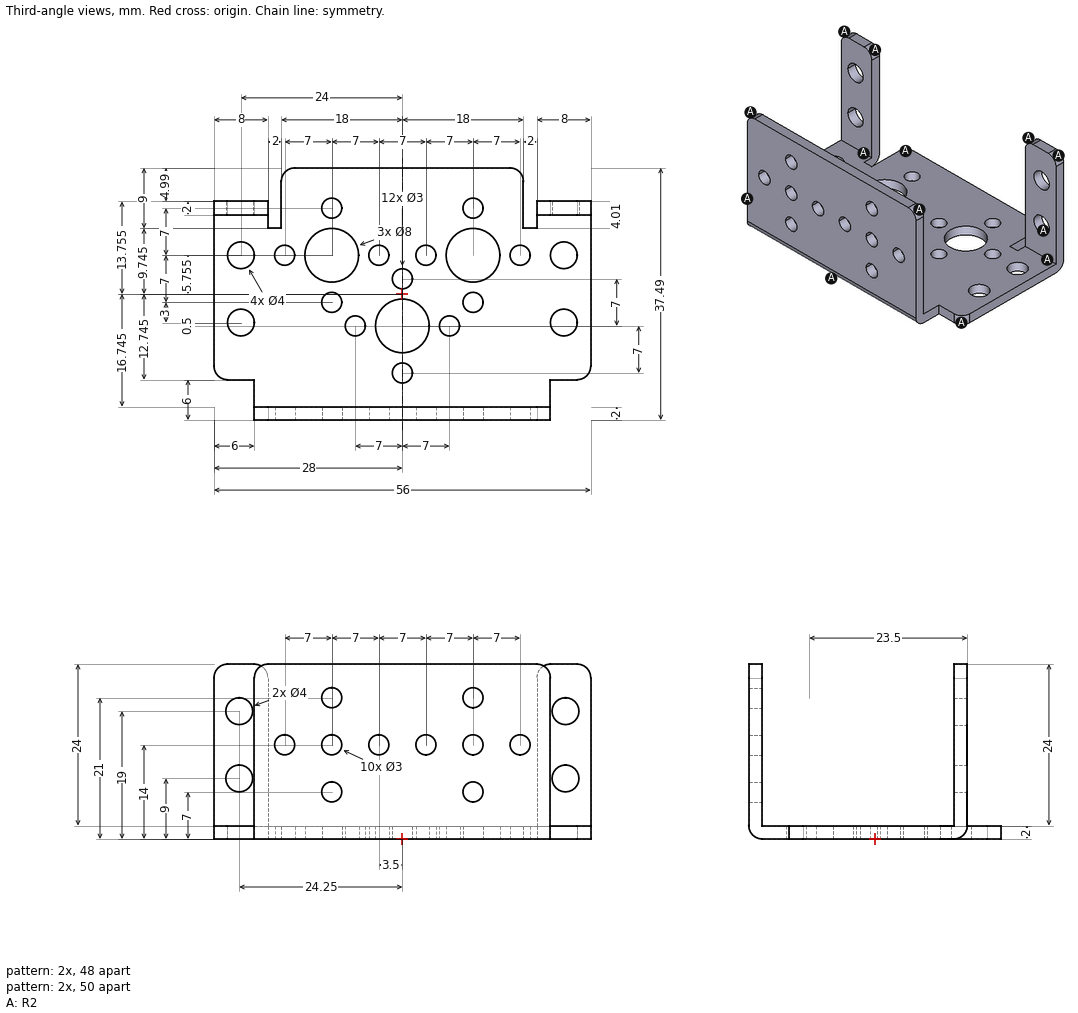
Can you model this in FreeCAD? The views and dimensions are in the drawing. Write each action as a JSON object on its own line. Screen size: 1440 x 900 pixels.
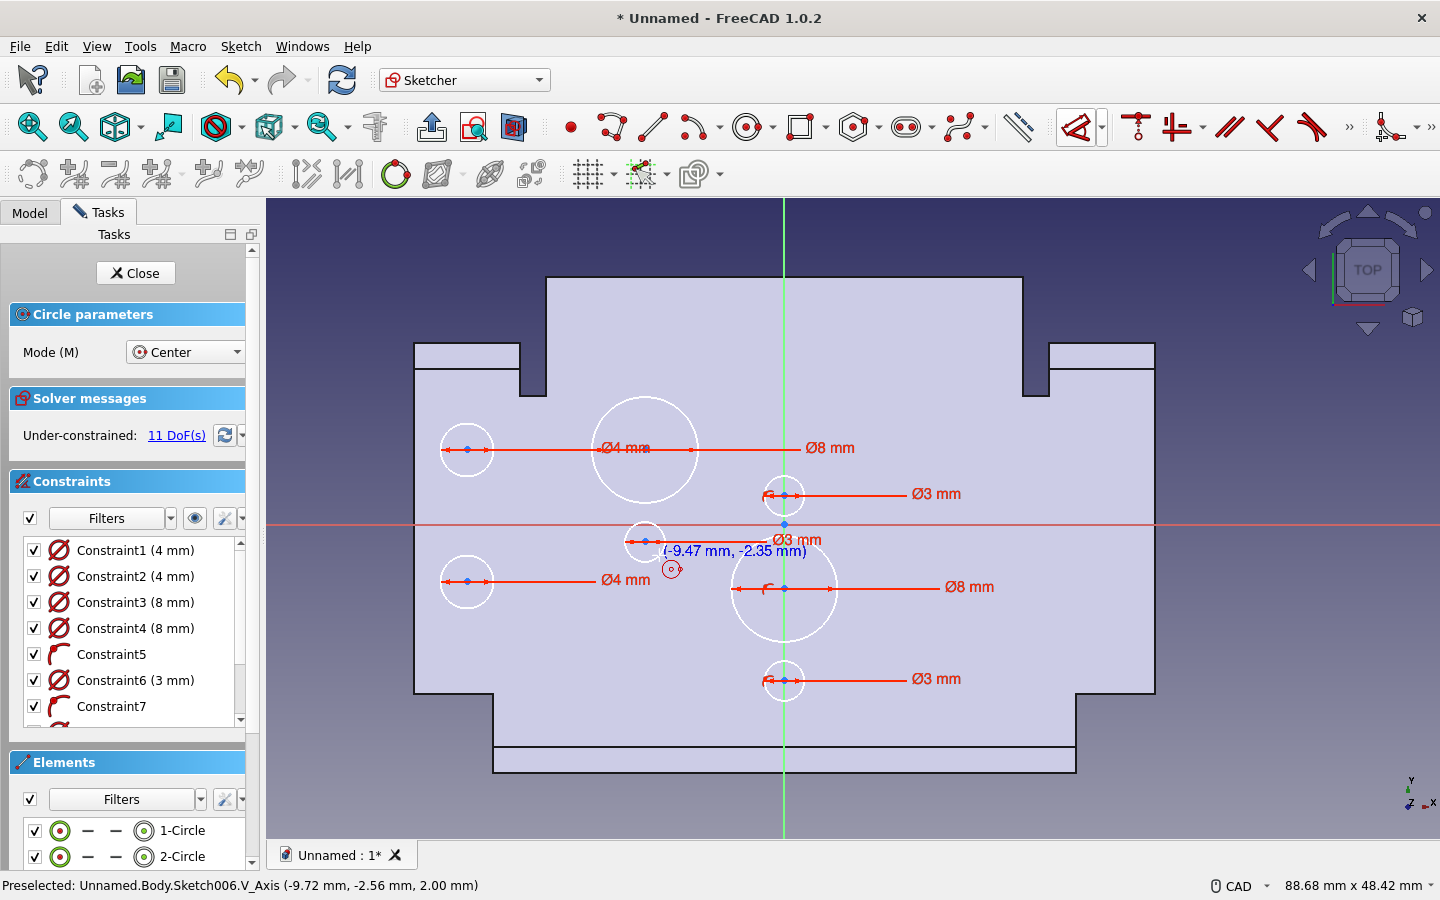
{"action": "left_click", "coordinate": [645, 356]}
{"action": "mouse_move", "coordinate": [659, 342]}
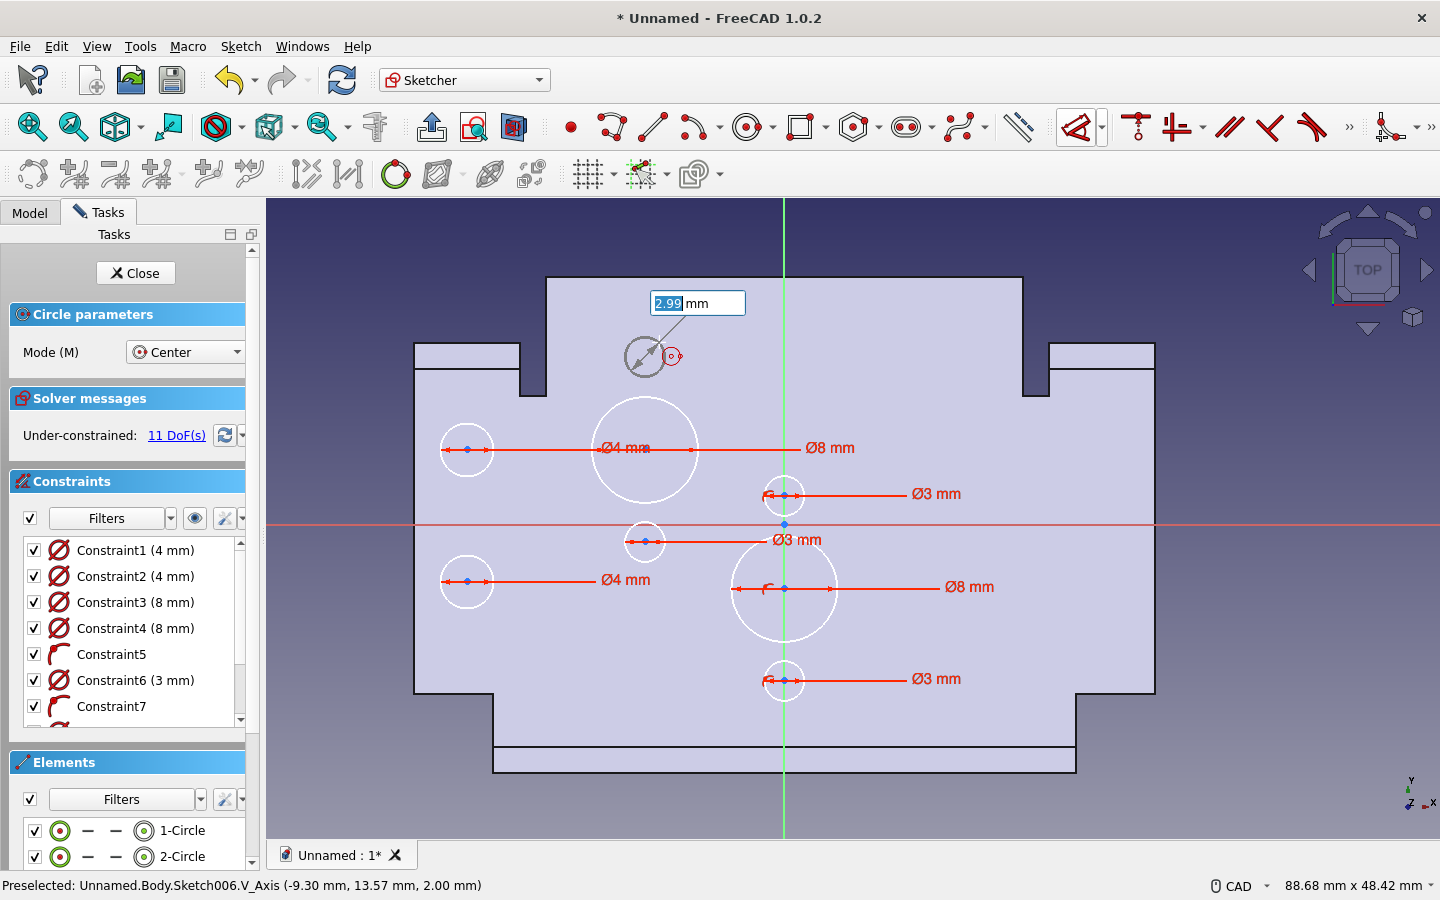
{"action": "type", "text": "3"}
{"action": "key", "text": "Return"}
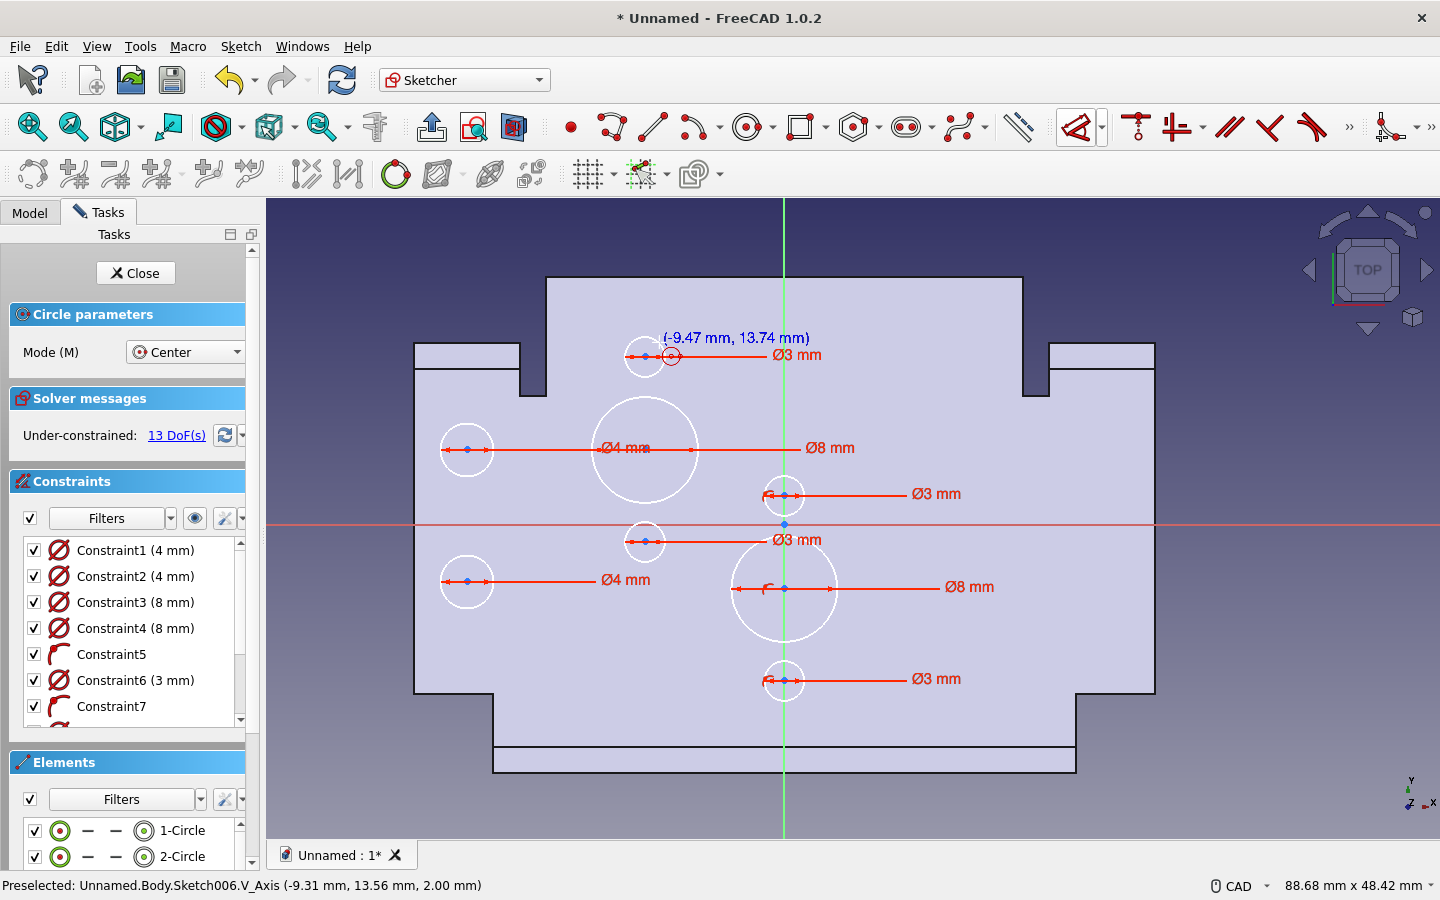
{"action": "left_click", "coordinate": [553, 449]}
{"action": "mouse_move", "coordinate": [567, 435]}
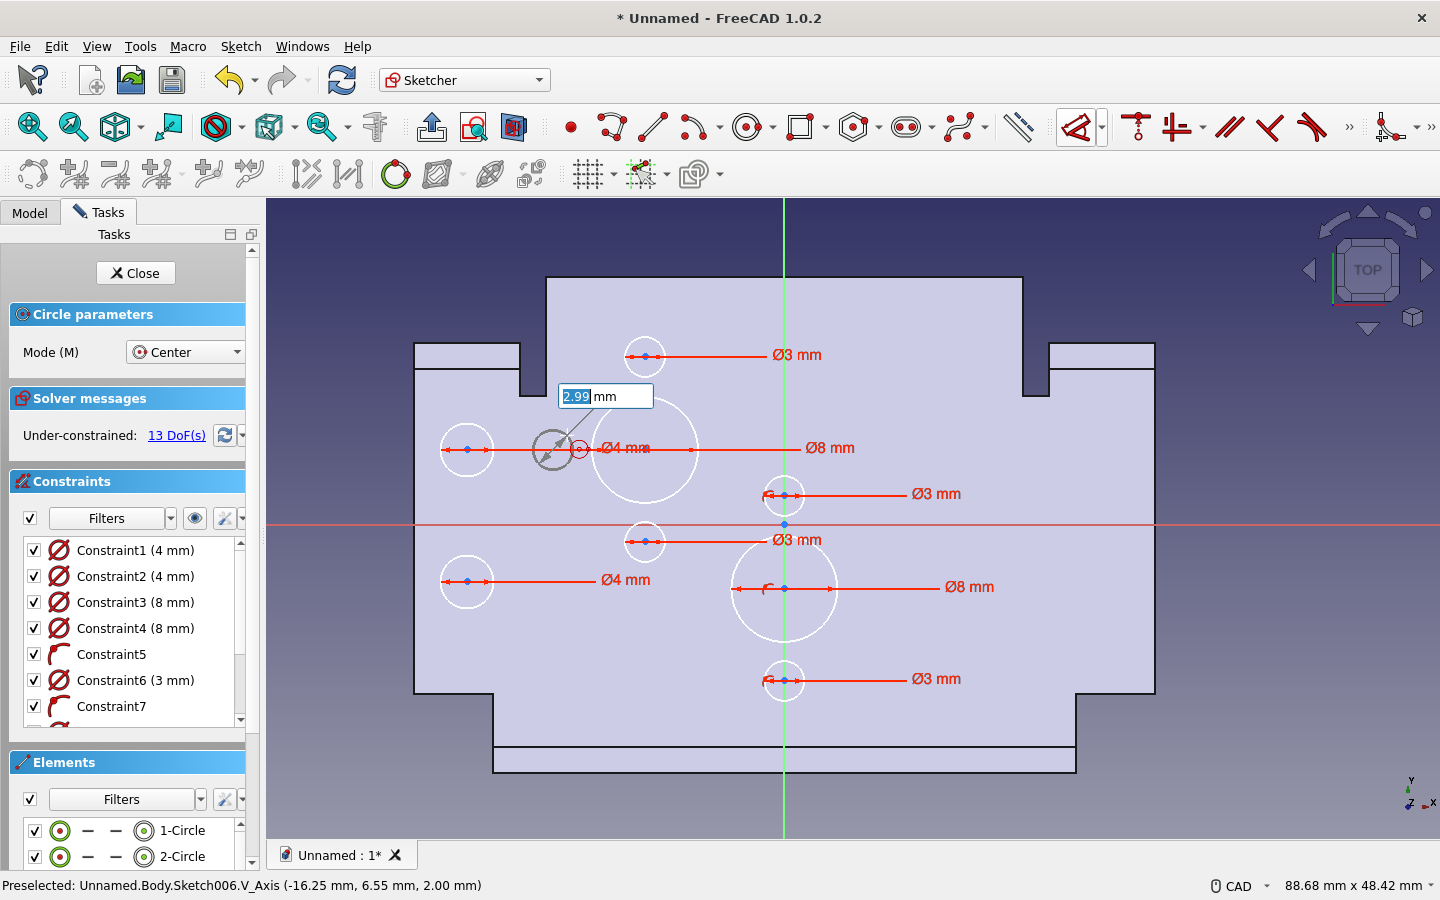
{"action": "type", "text": "3"}
{"action": "key", "text": "Return"}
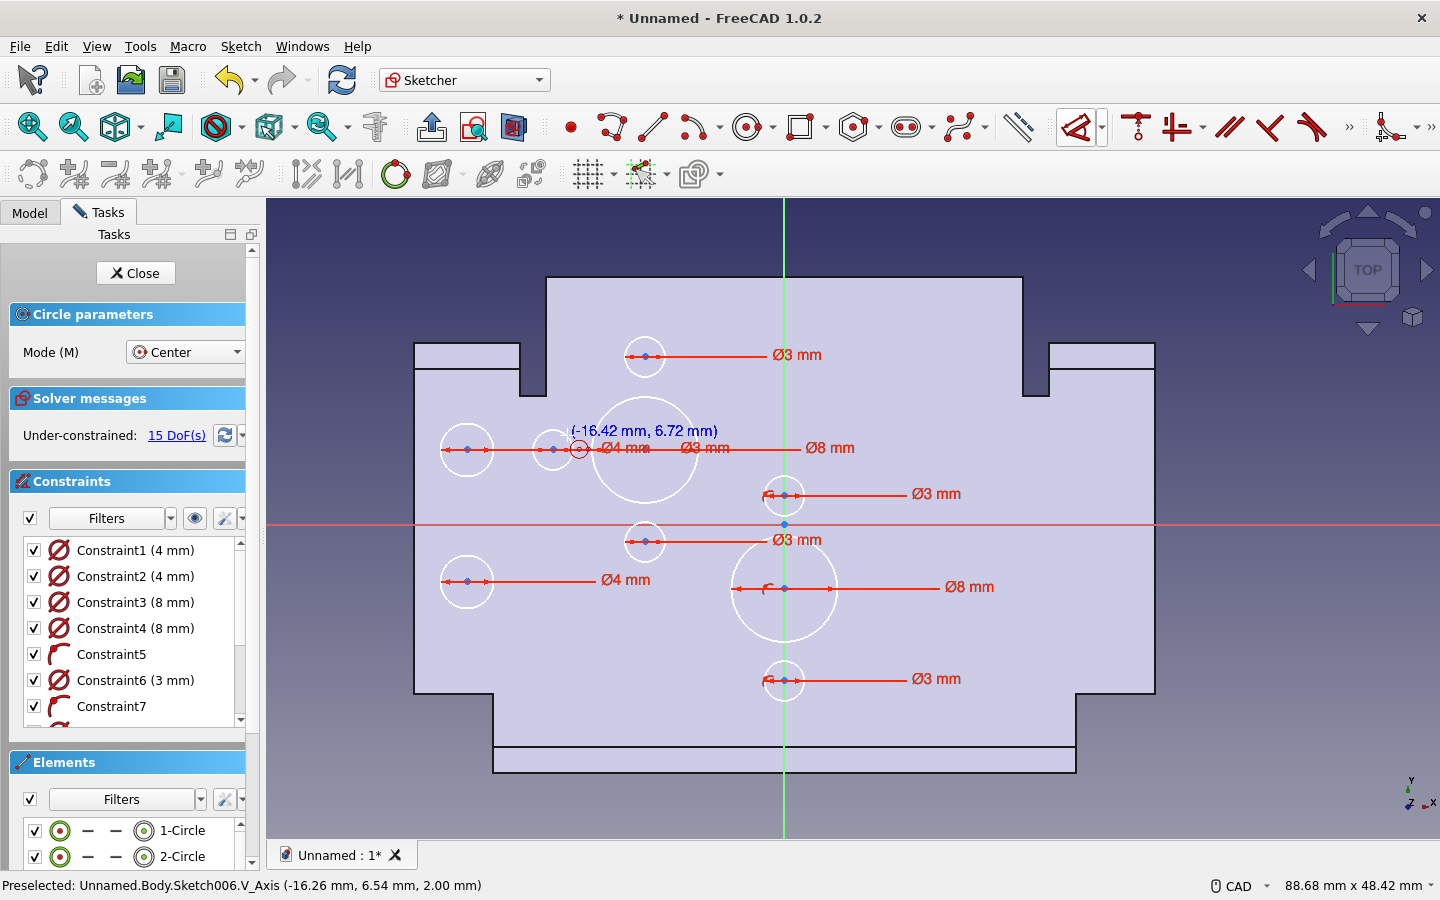
{"action": "left_click", "coordinate": [738, 449]}
{"action": "mouse_move", "coordinate": [752, 435]}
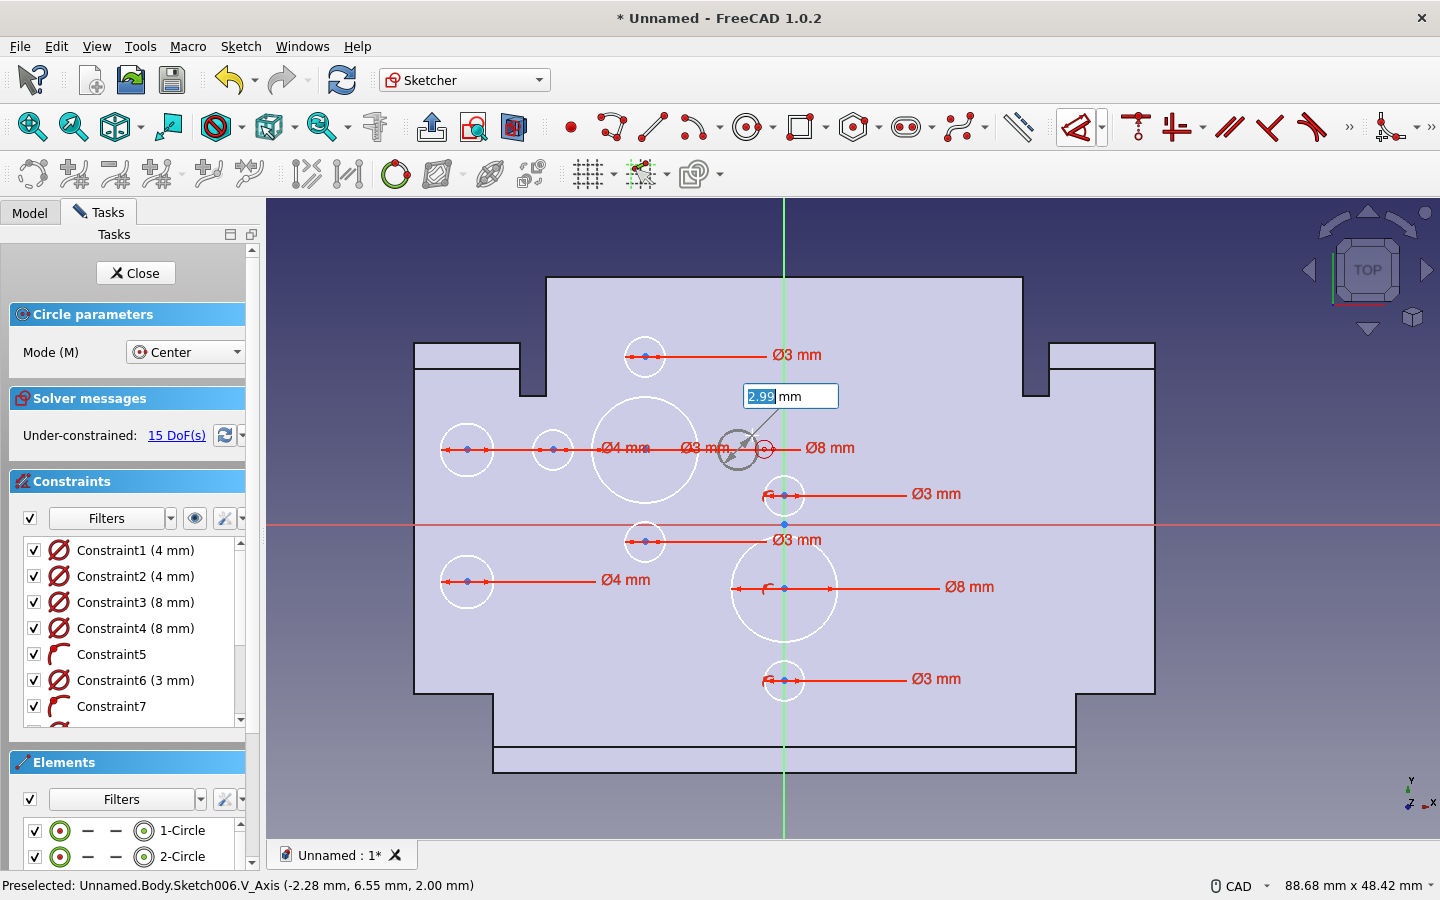
{"action": "type", "text": "3"}
{"action": "key", "text": "Return"}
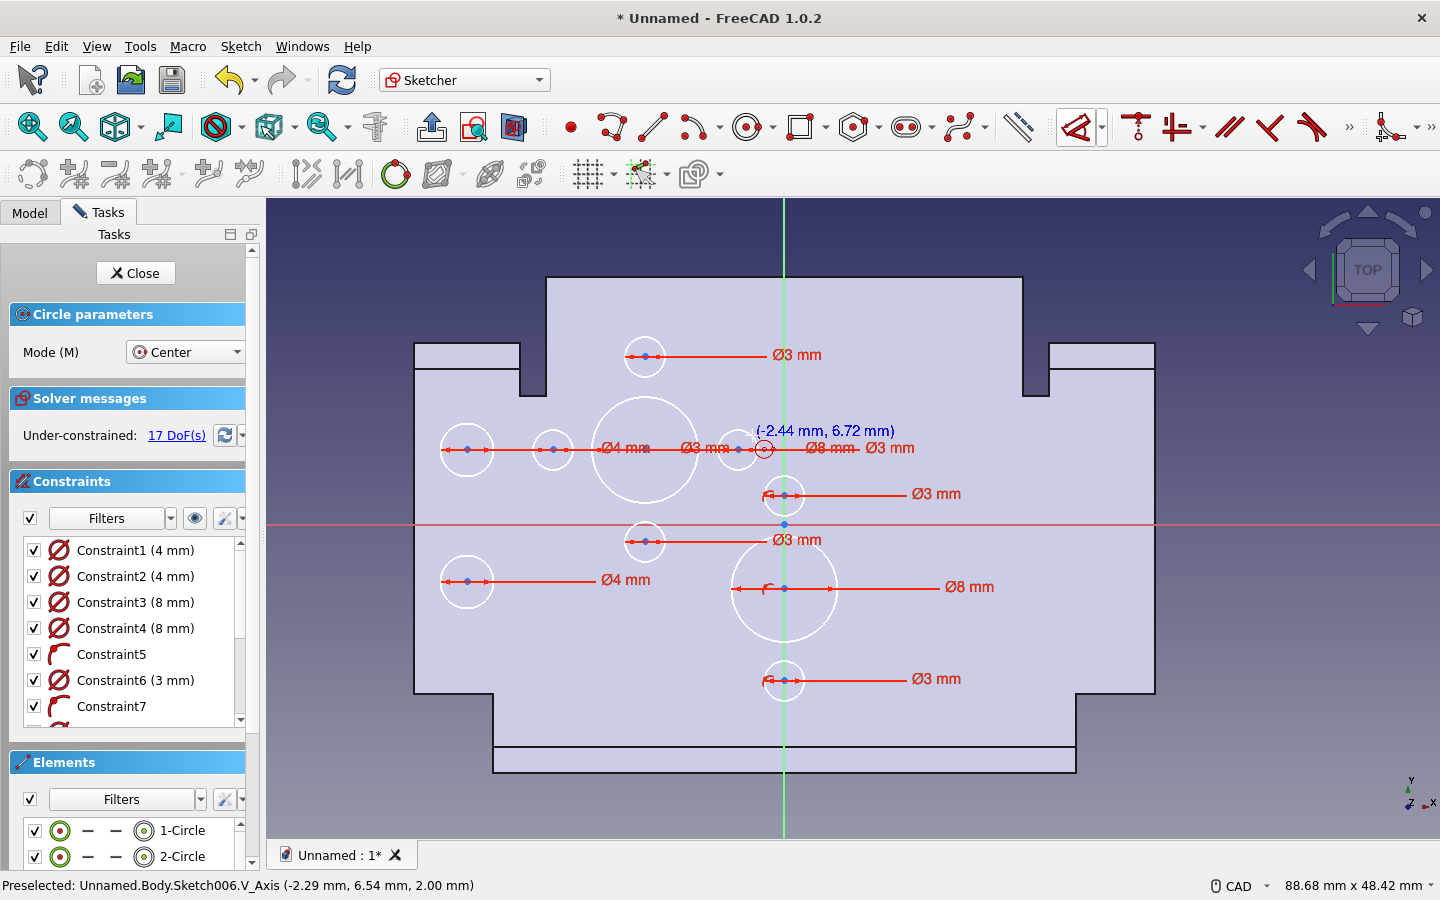
{"action": "left_click", "coordinate": [692, 588]}
{"action": "mouse_move", "coordinate": [706, 574]}